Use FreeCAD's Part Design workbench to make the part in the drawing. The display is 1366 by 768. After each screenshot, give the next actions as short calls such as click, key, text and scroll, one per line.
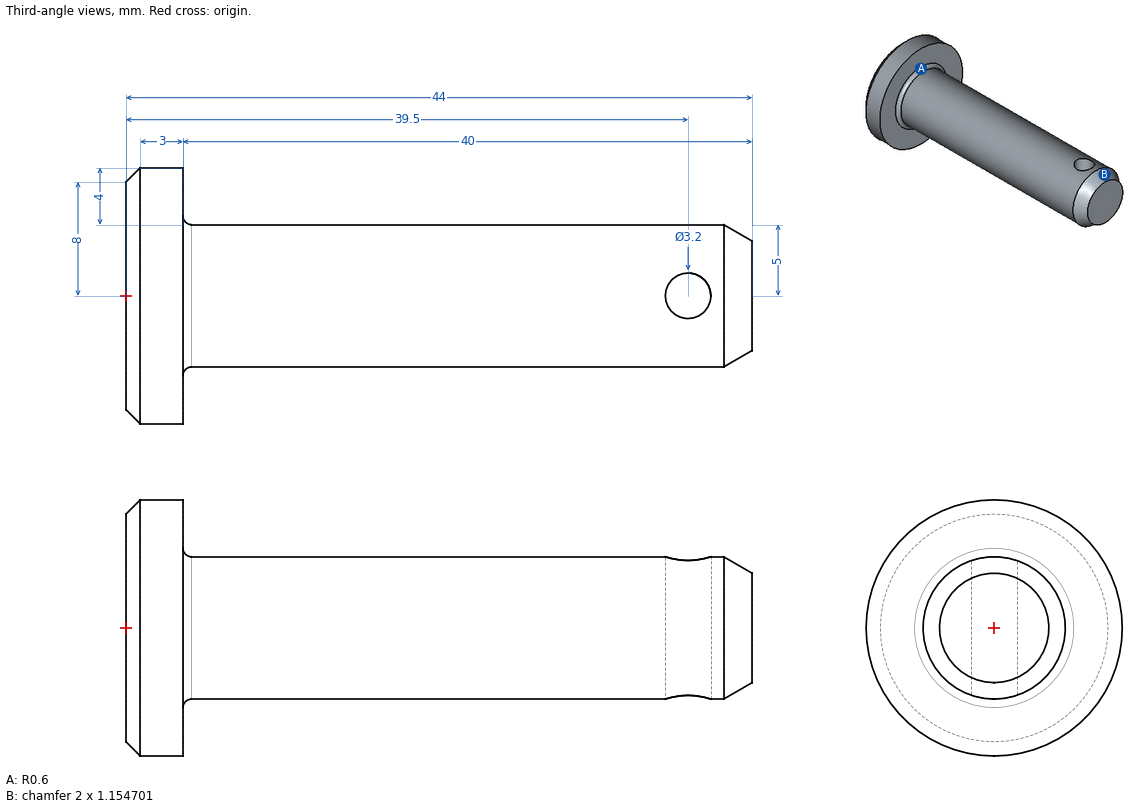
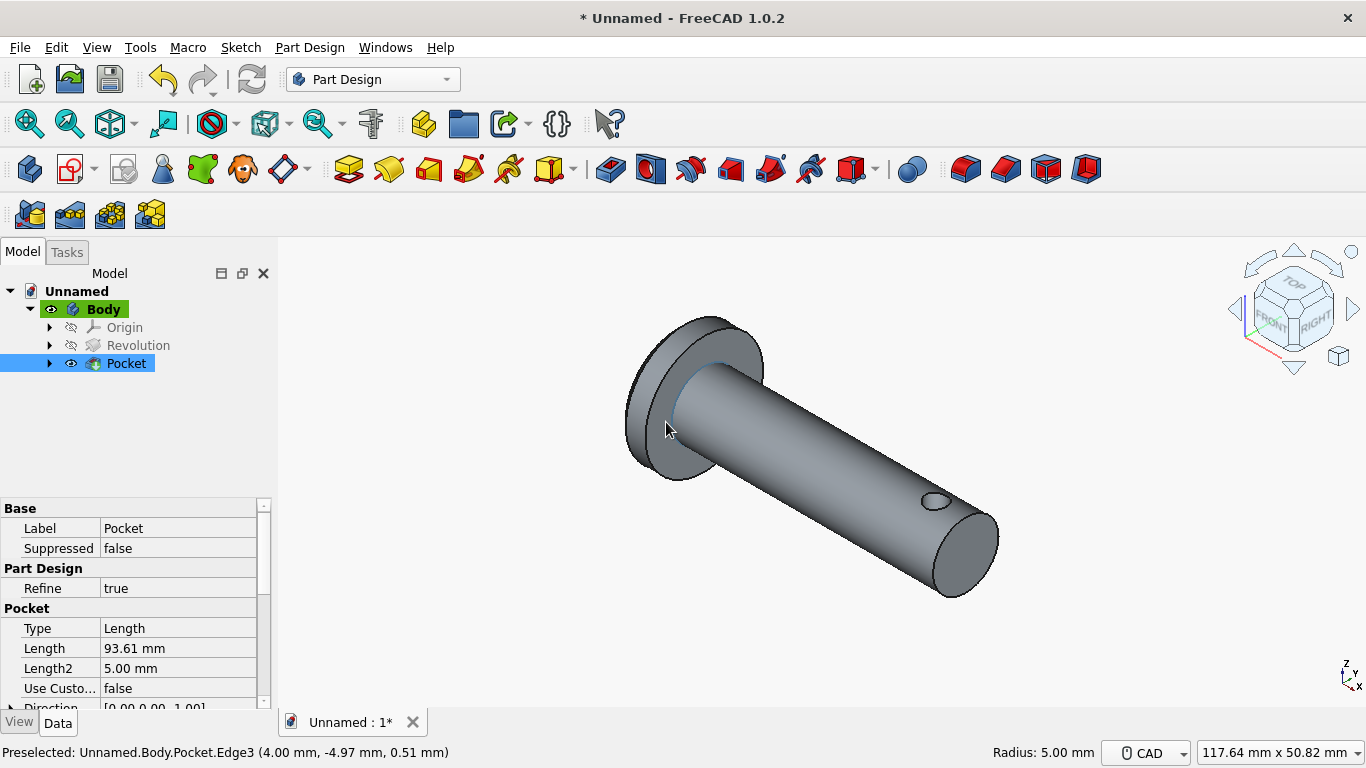
click(966, 170)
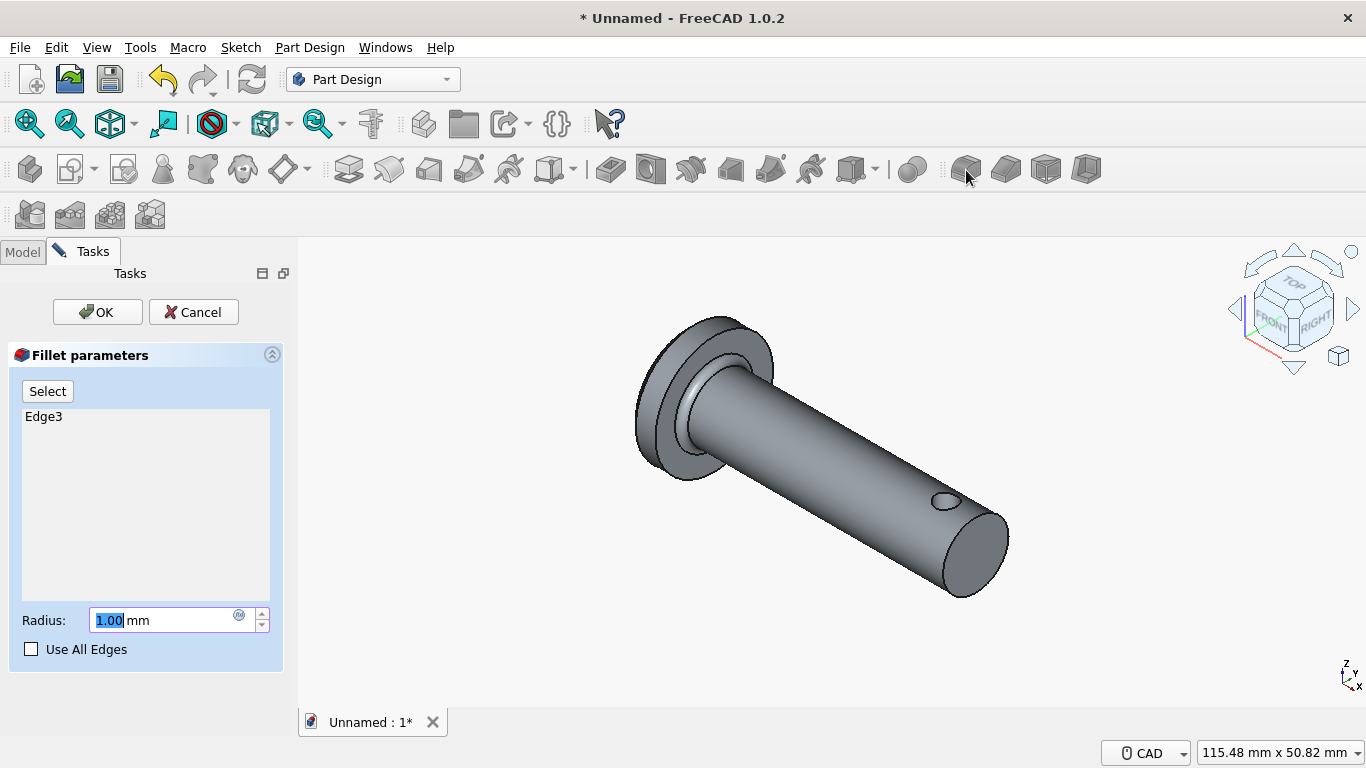
text(0.6)
key(Tab)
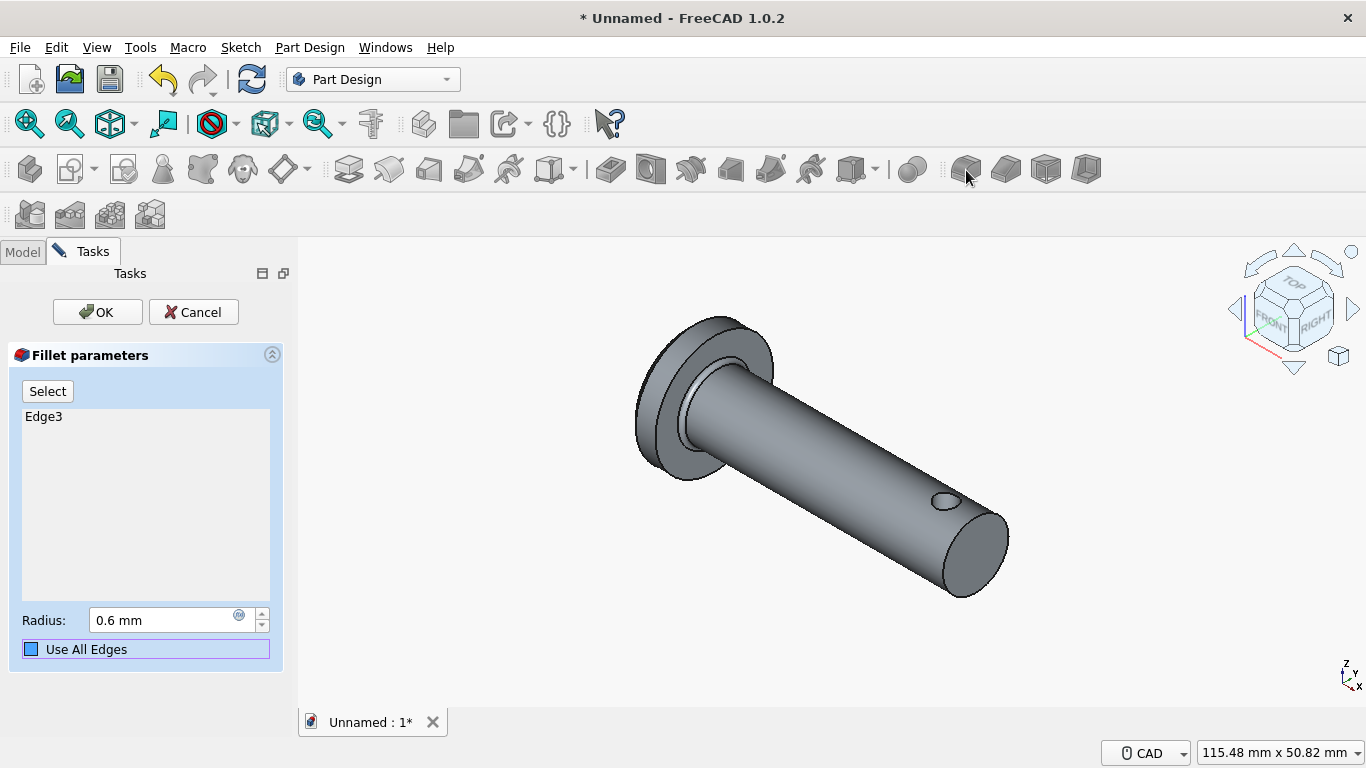
click(98, 312)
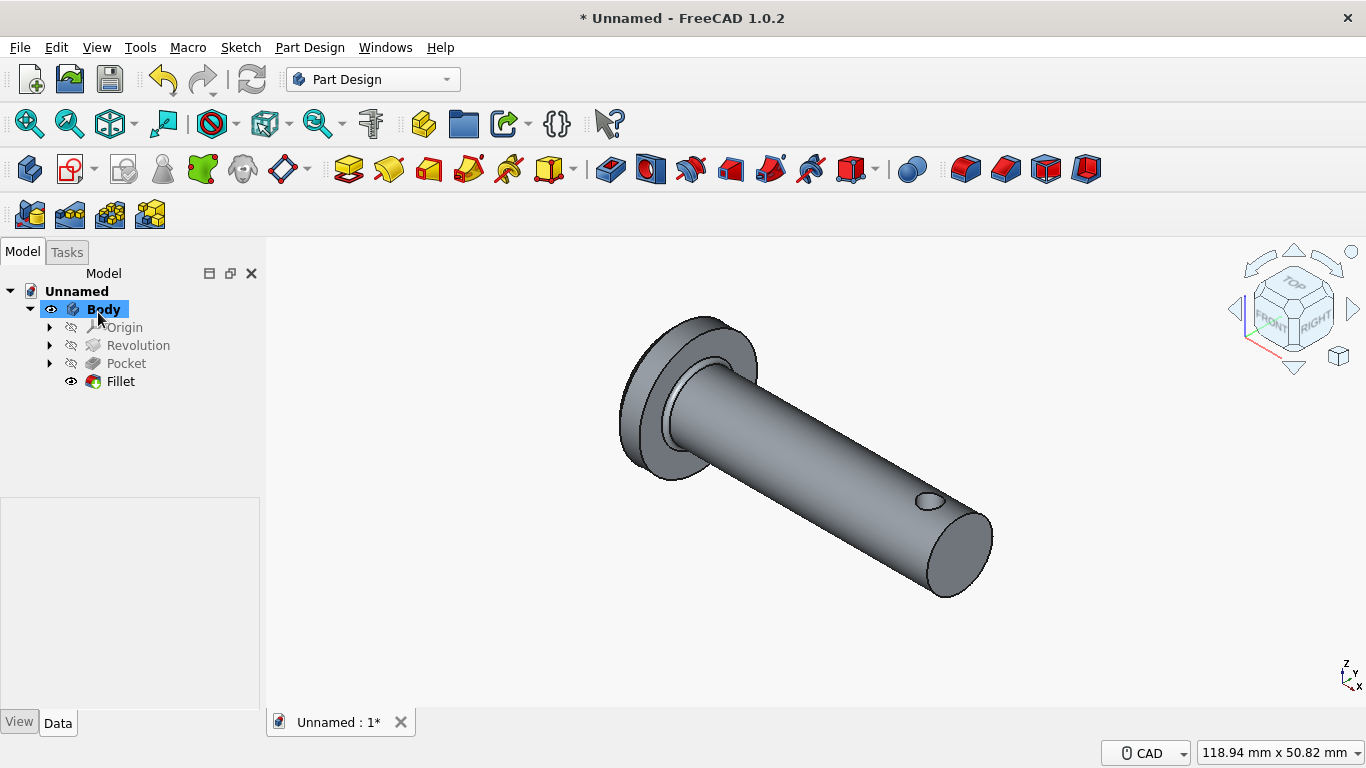
click(927, 573)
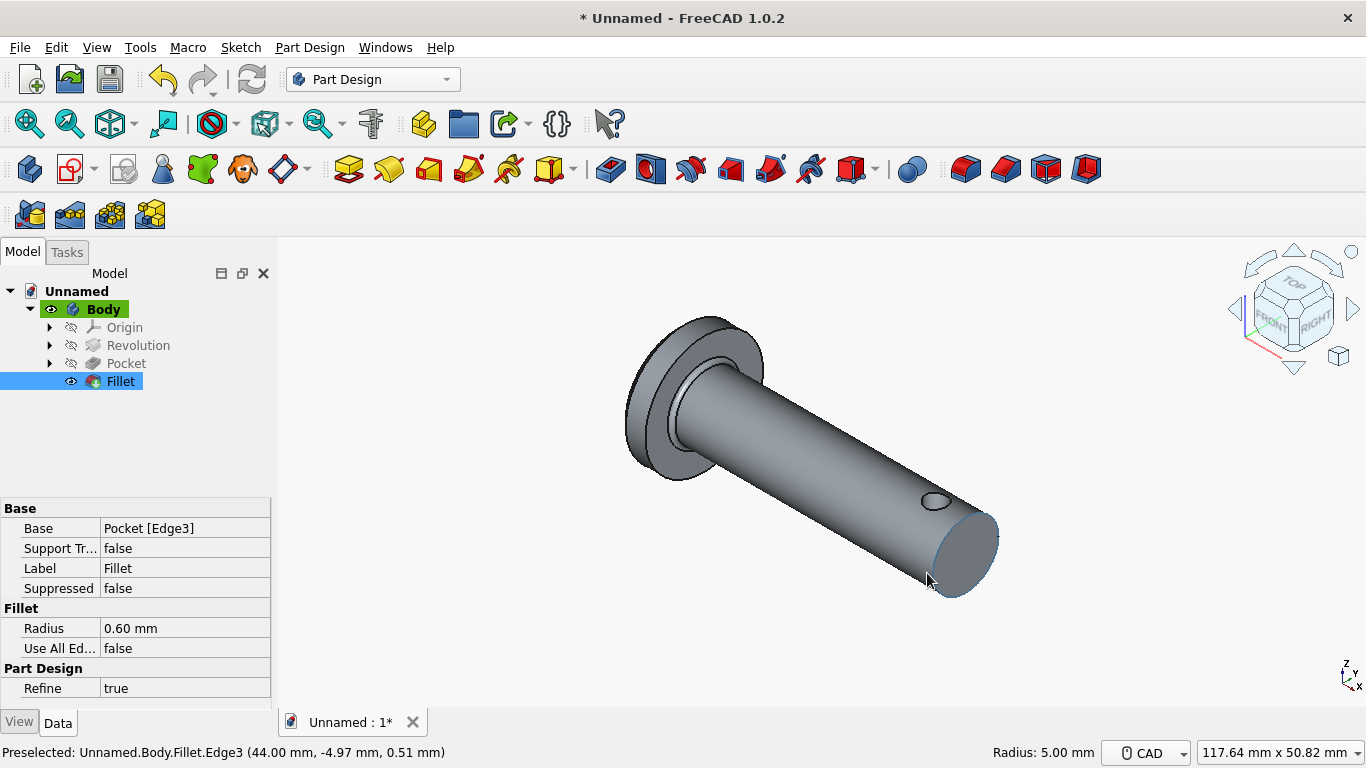
click(1006, 170)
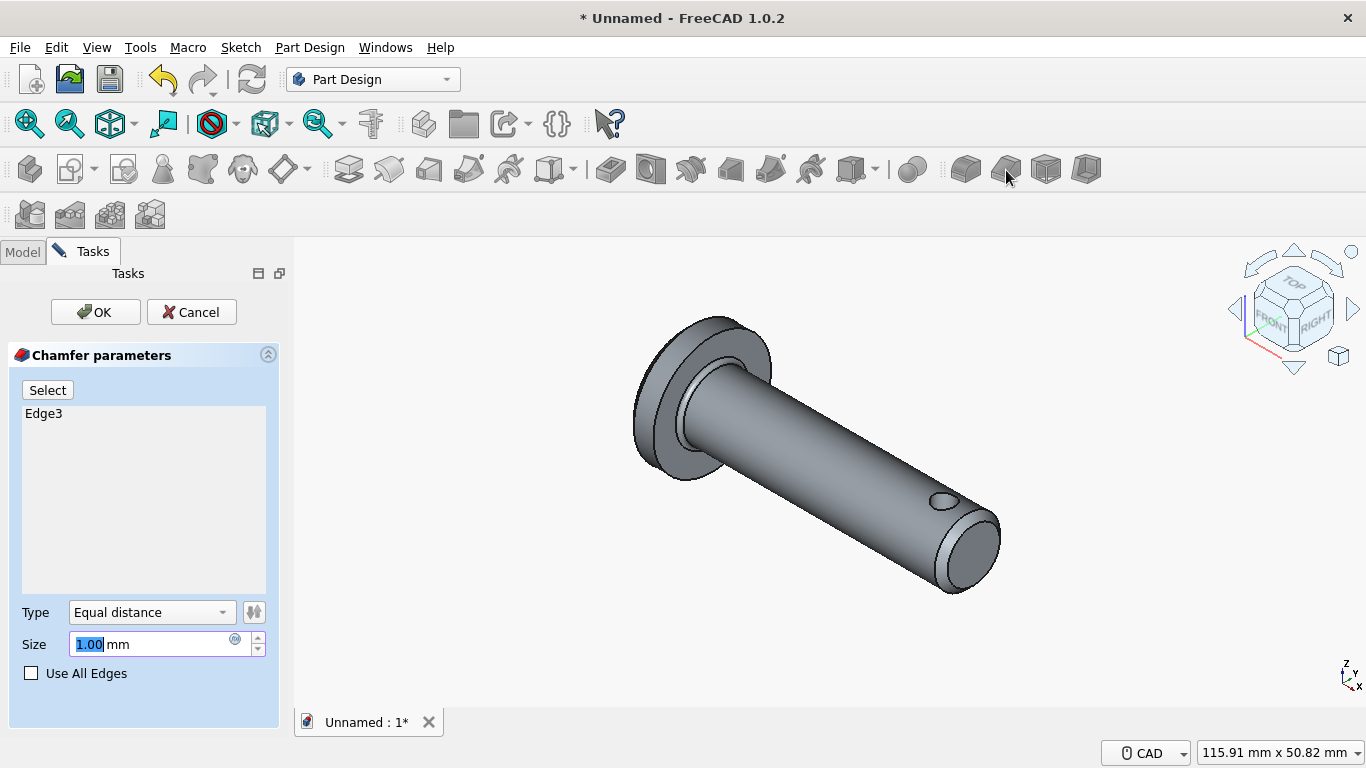
text(2)
key(Tab)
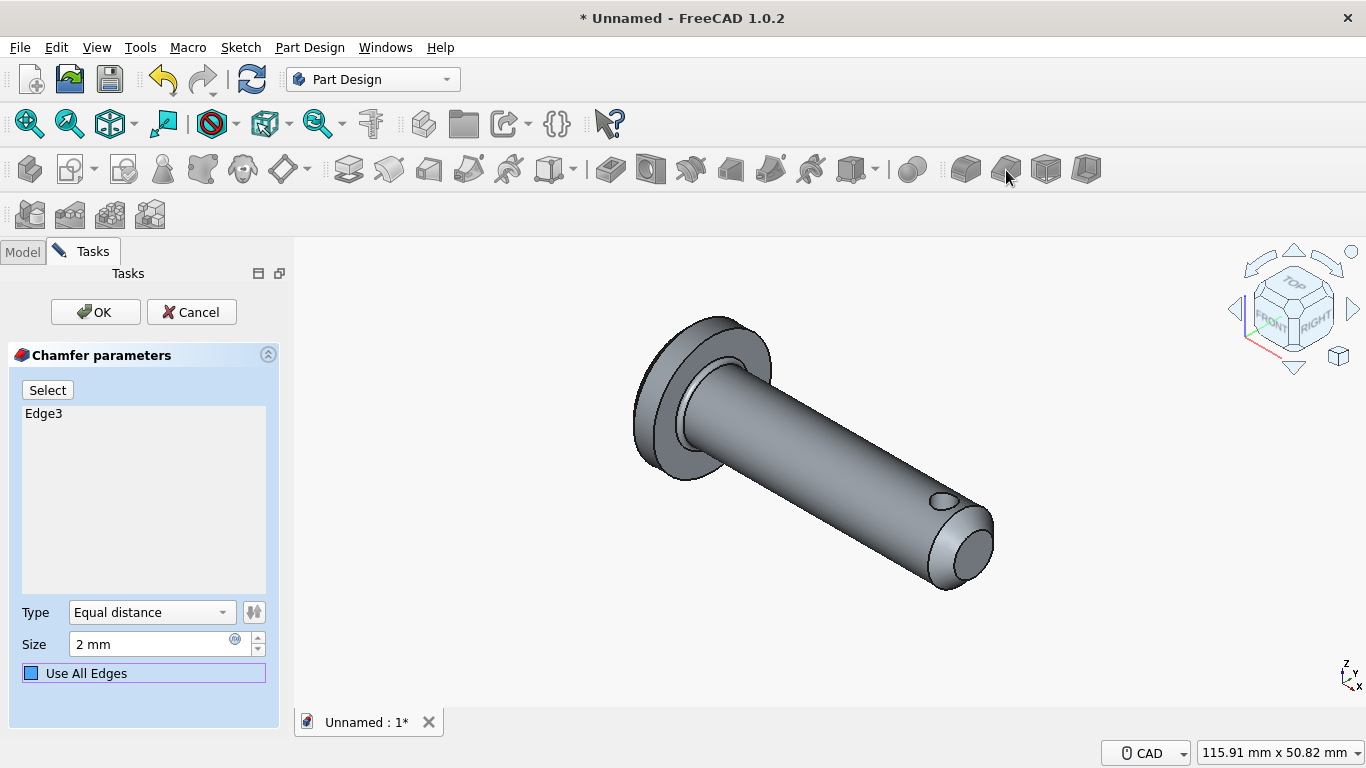
click(153, 612)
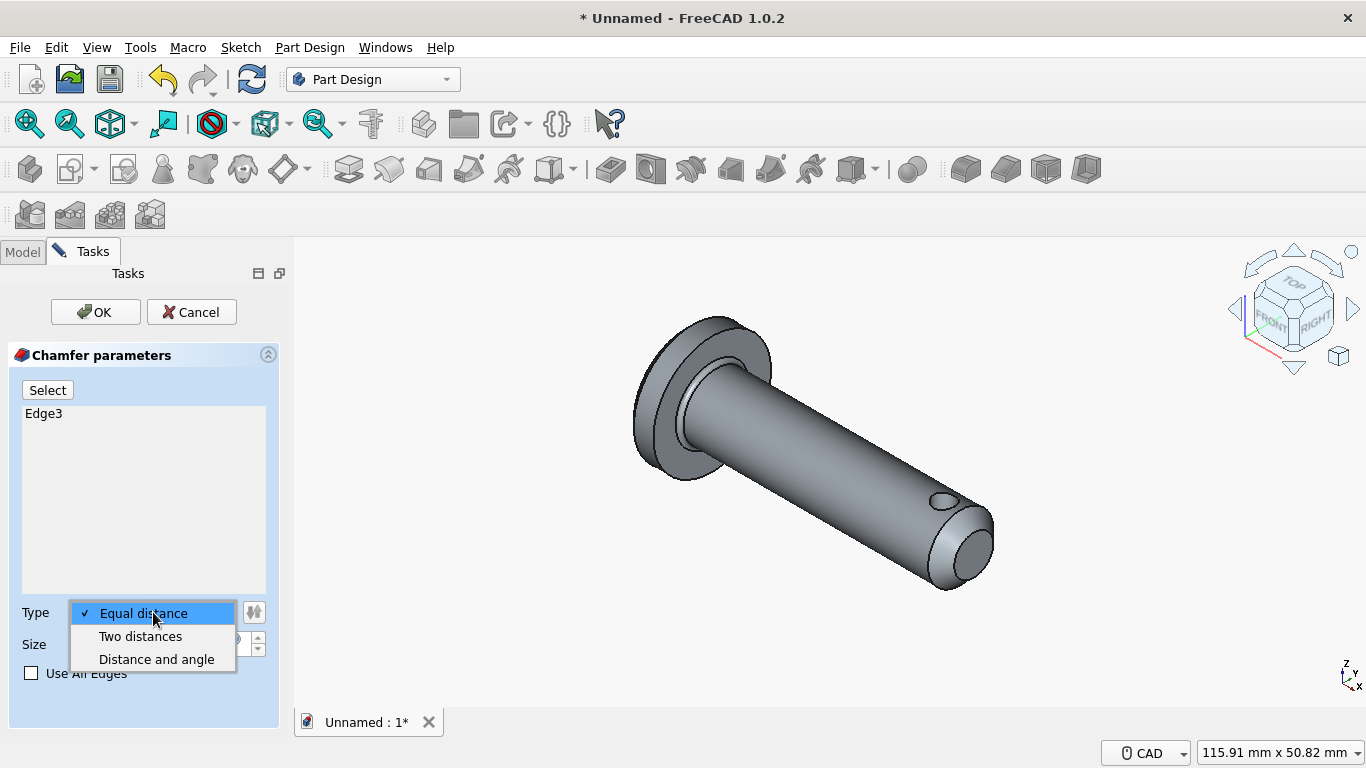
click(152, 636)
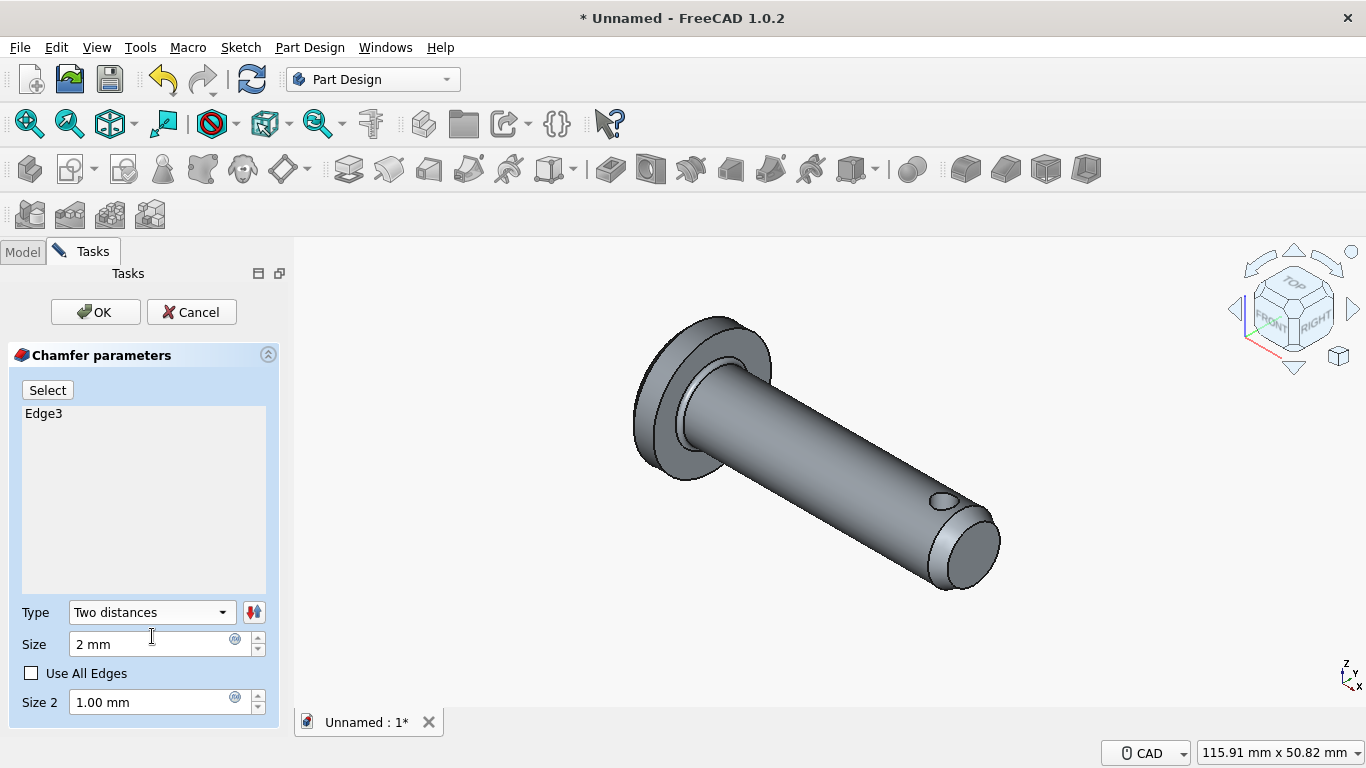
triple_click(160, 702)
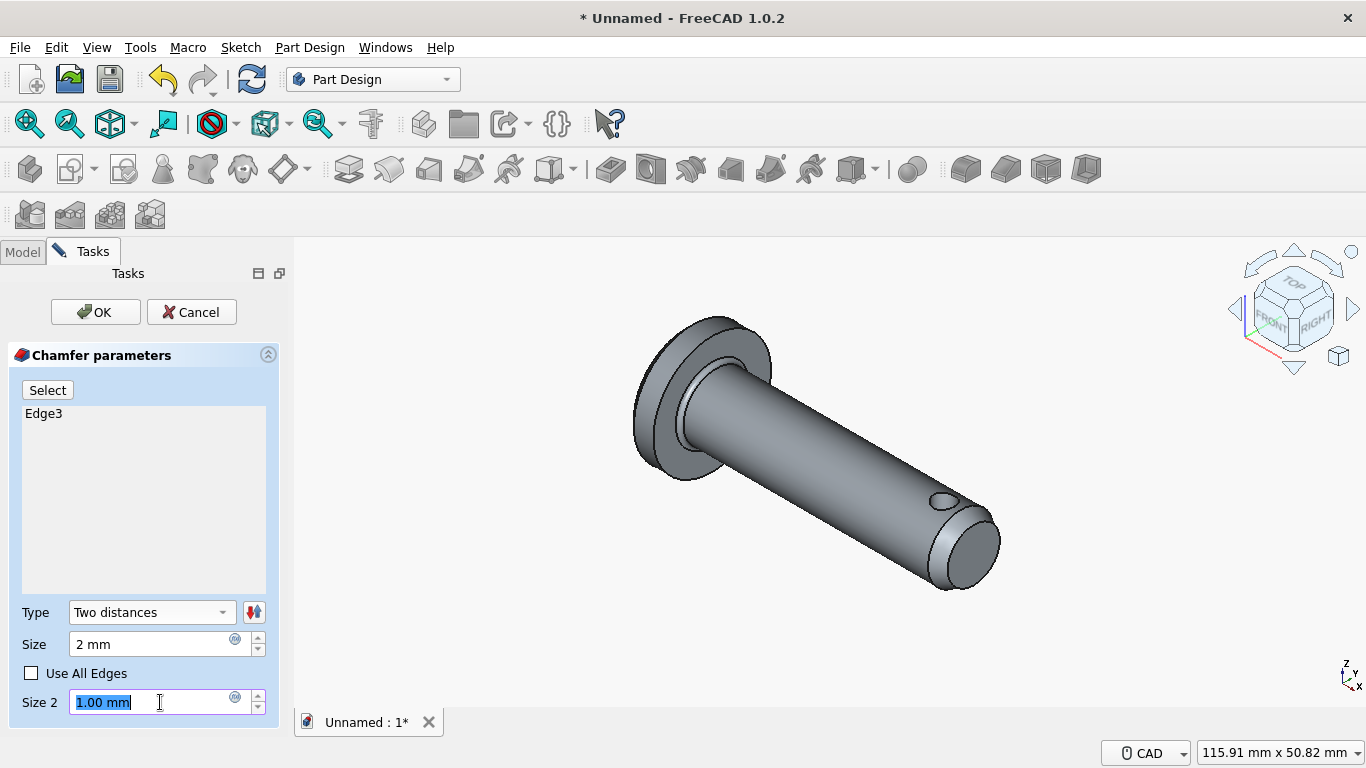
text(1.154701)
key(Tab)